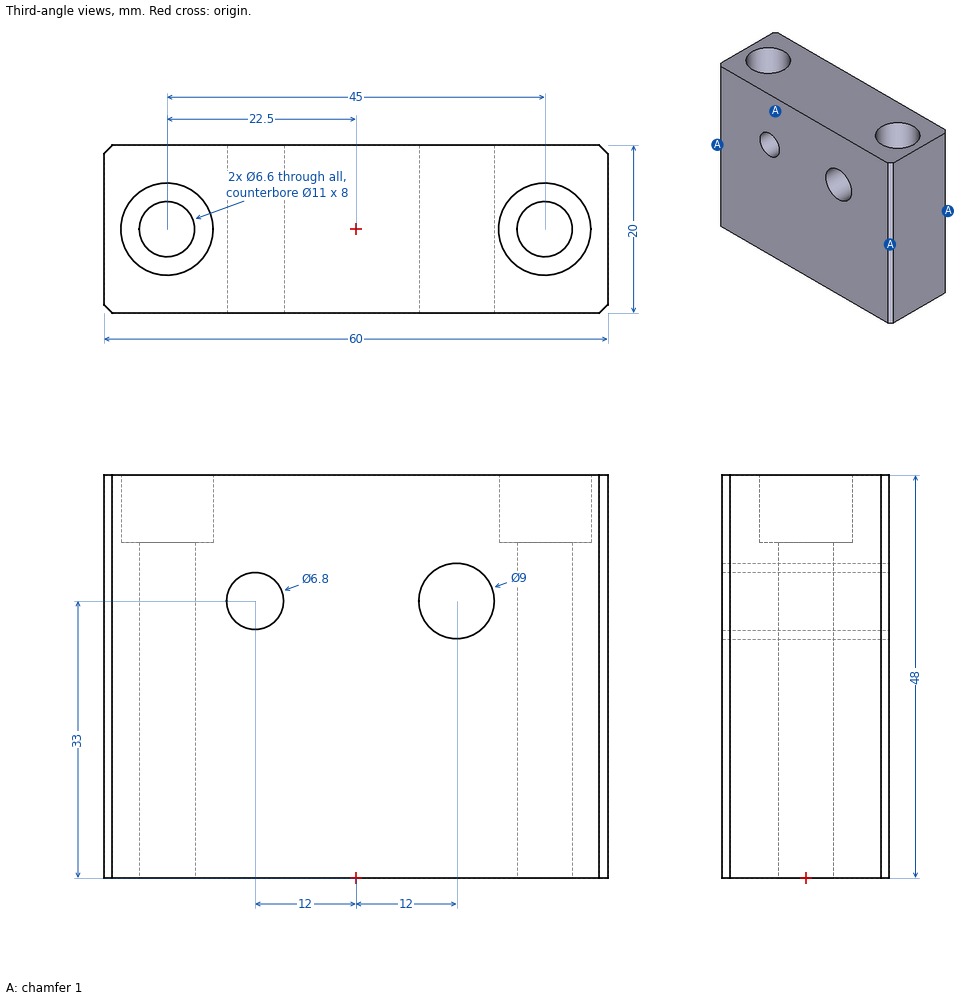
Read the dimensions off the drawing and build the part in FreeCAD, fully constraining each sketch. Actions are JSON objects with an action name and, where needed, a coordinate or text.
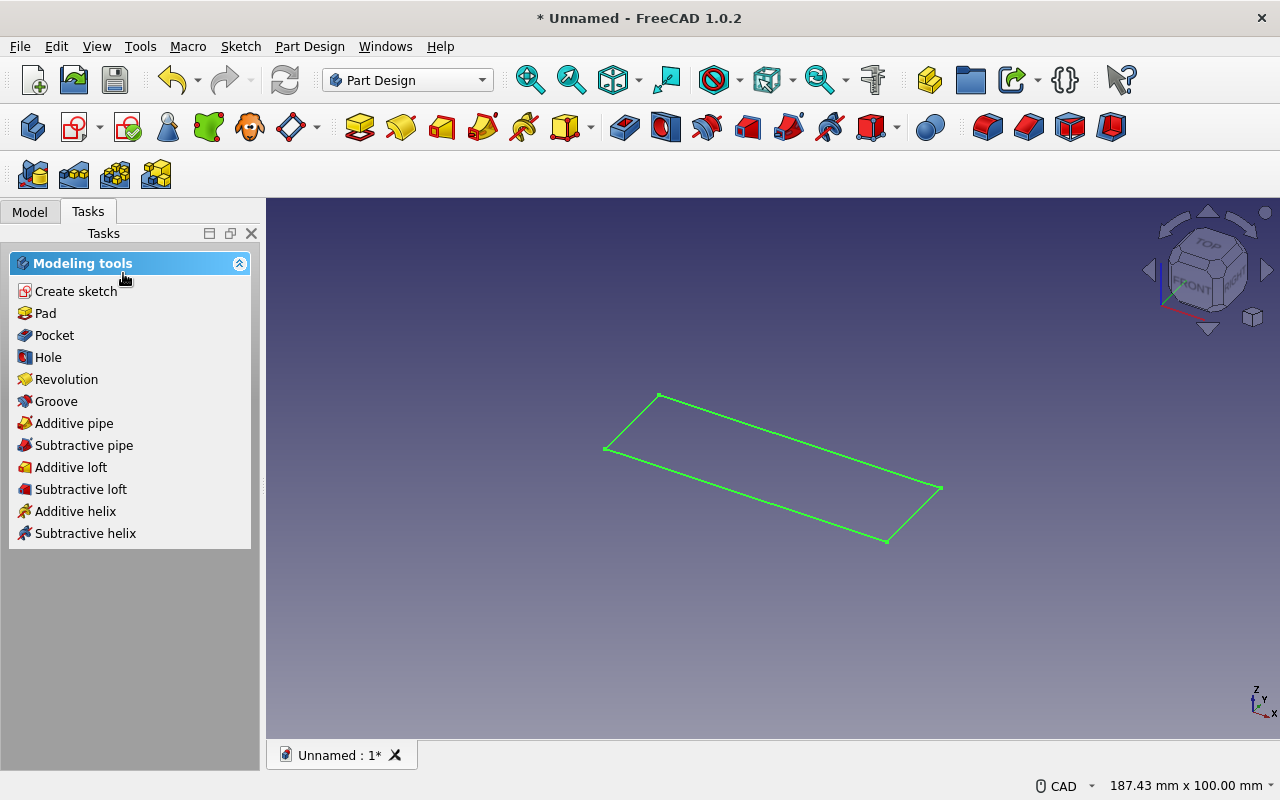
{"action": "left_click", "coordinate": [360, 128]}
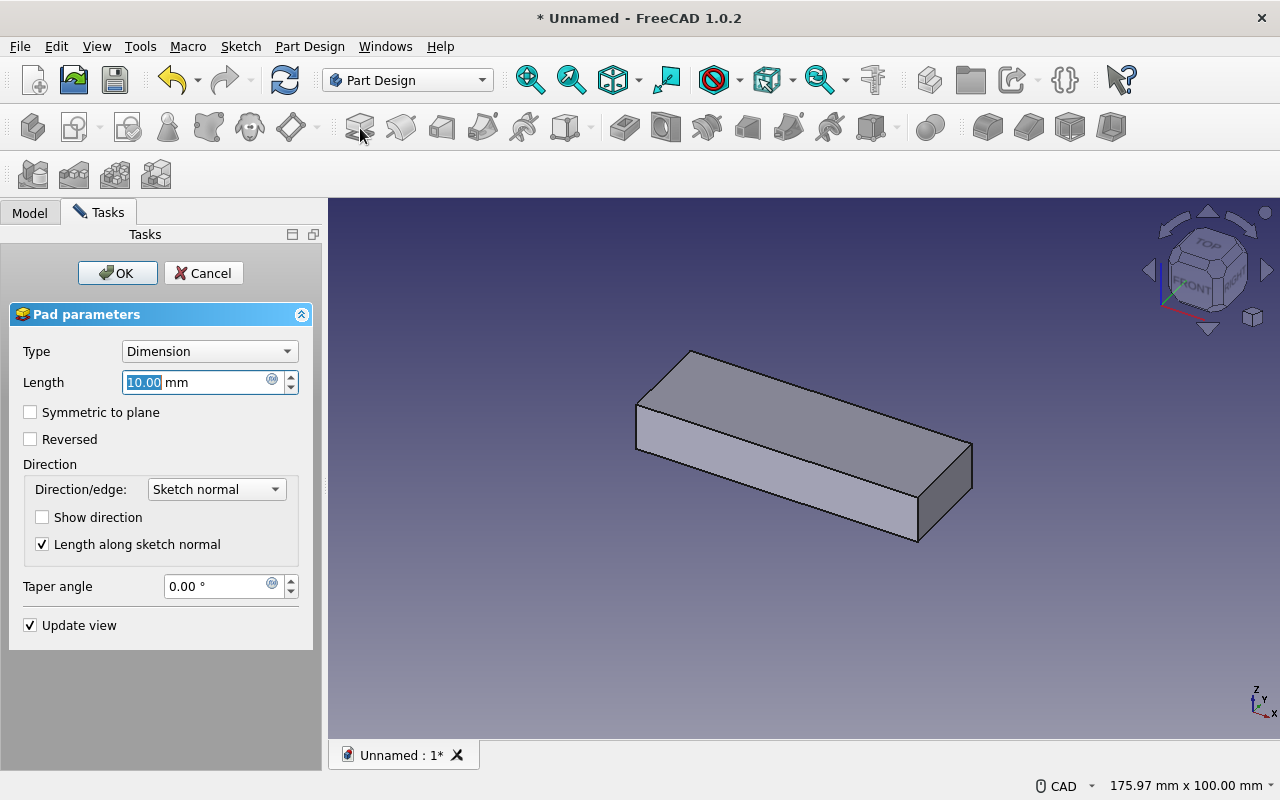
{"action": "type", "text": "48"}
{"action": "key", "text": "Tab"}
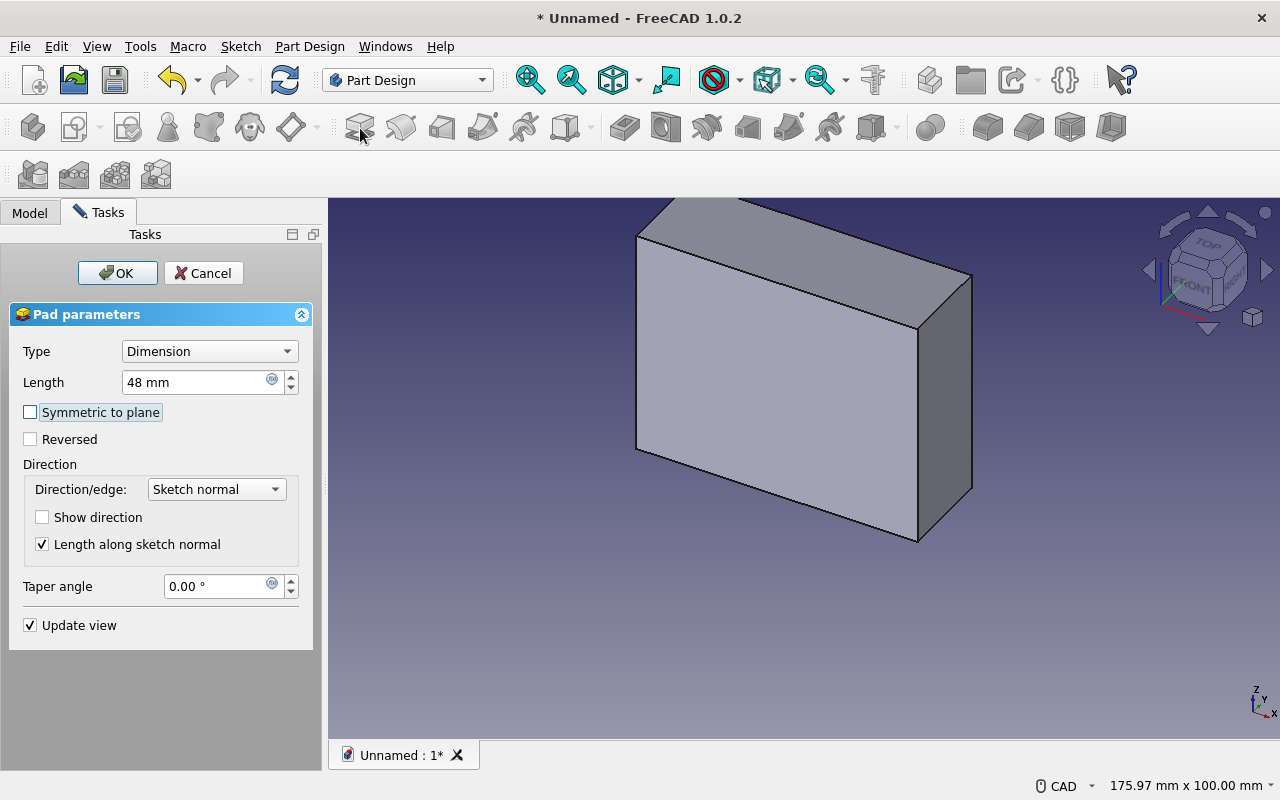
{"action": "left_click", "coordinate": [118, 273]}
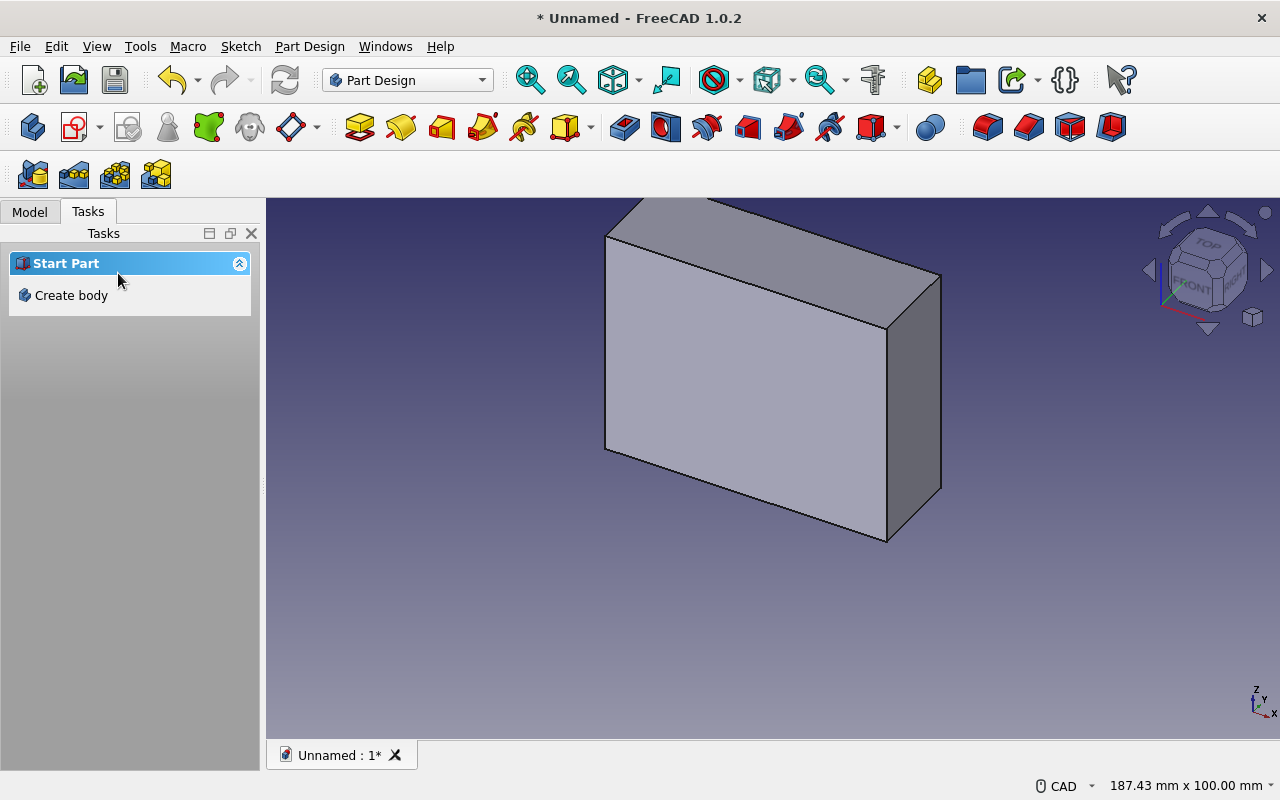
{"action": "left_click", "coordinate": [531, 80]}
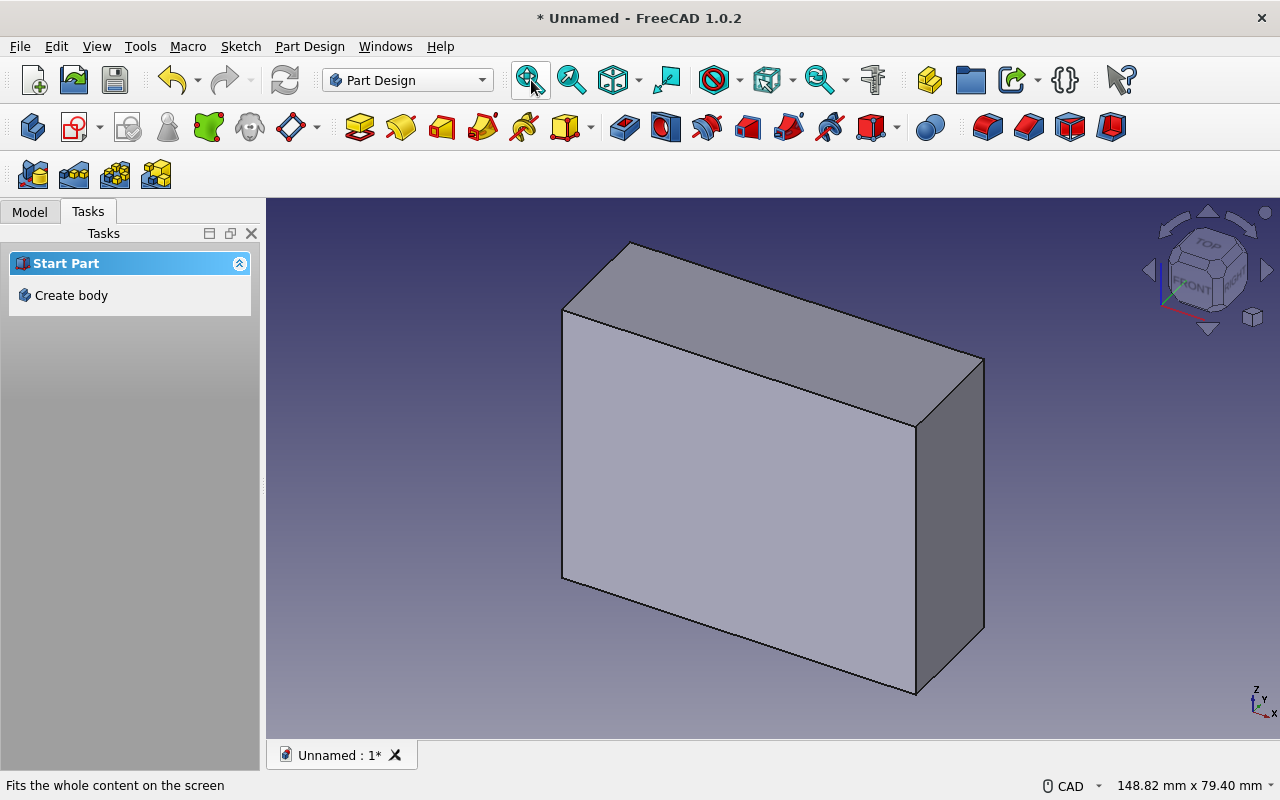
{"action": "left_click", "coordinate": [874, 367]}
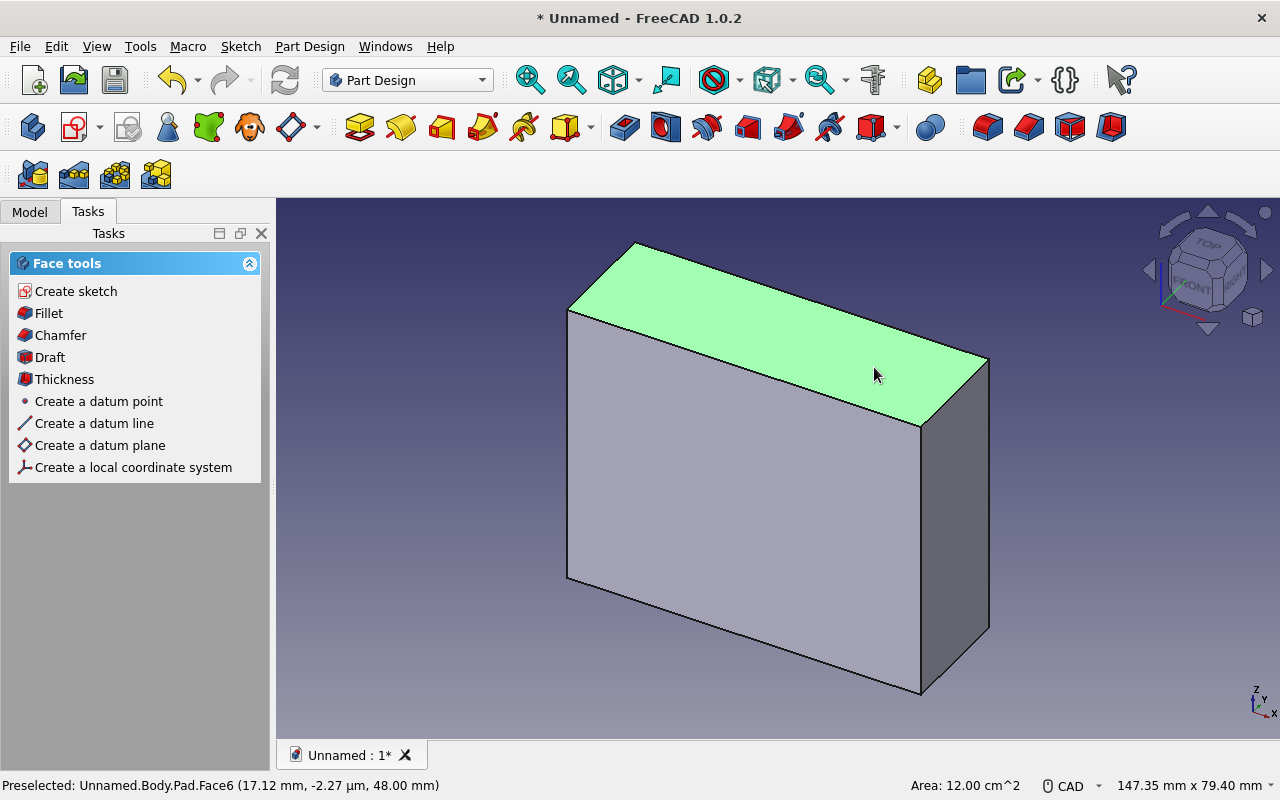
{"action": "left_click", "coordinate": [74, 128]}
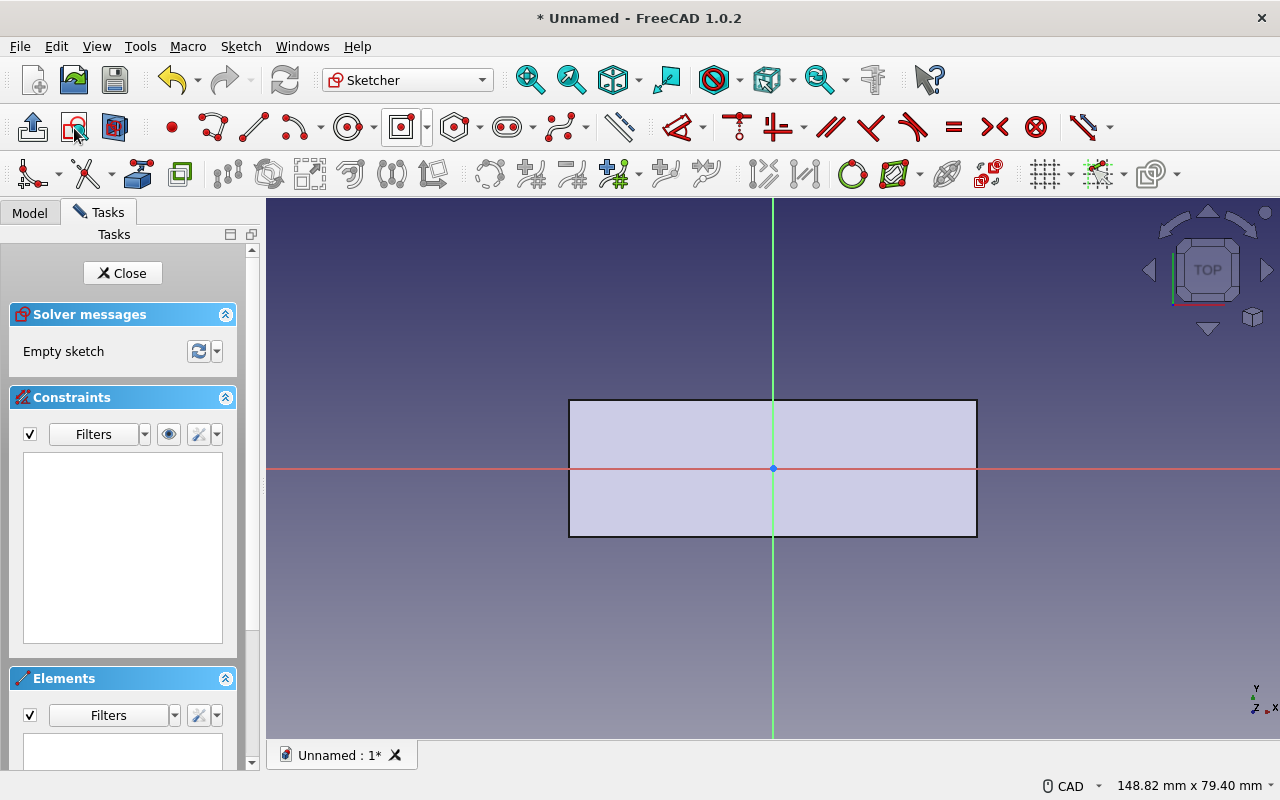
{"action": "scroll", "coordinate": [912, 469], "scroll_direction": "up", "scroll_amount": 2}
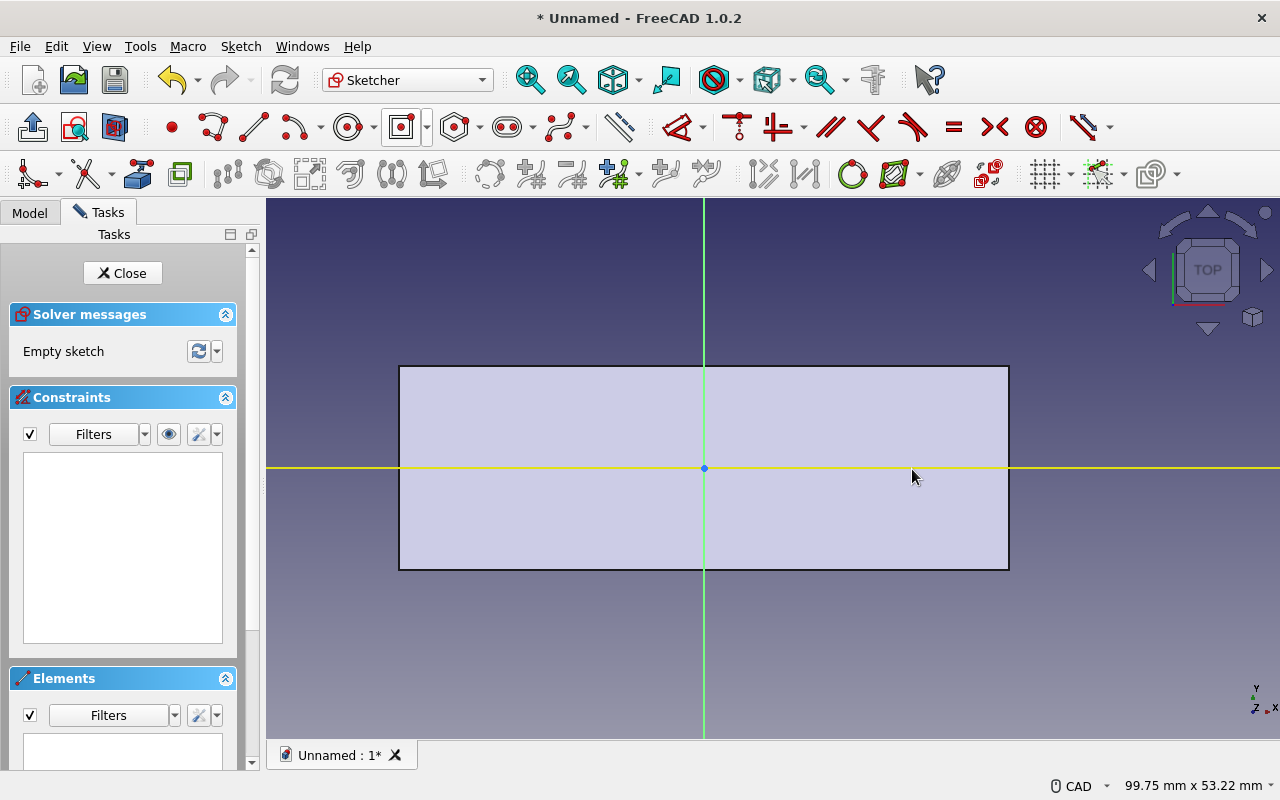
{"action": "left_click", "coordinate": [348, 128]}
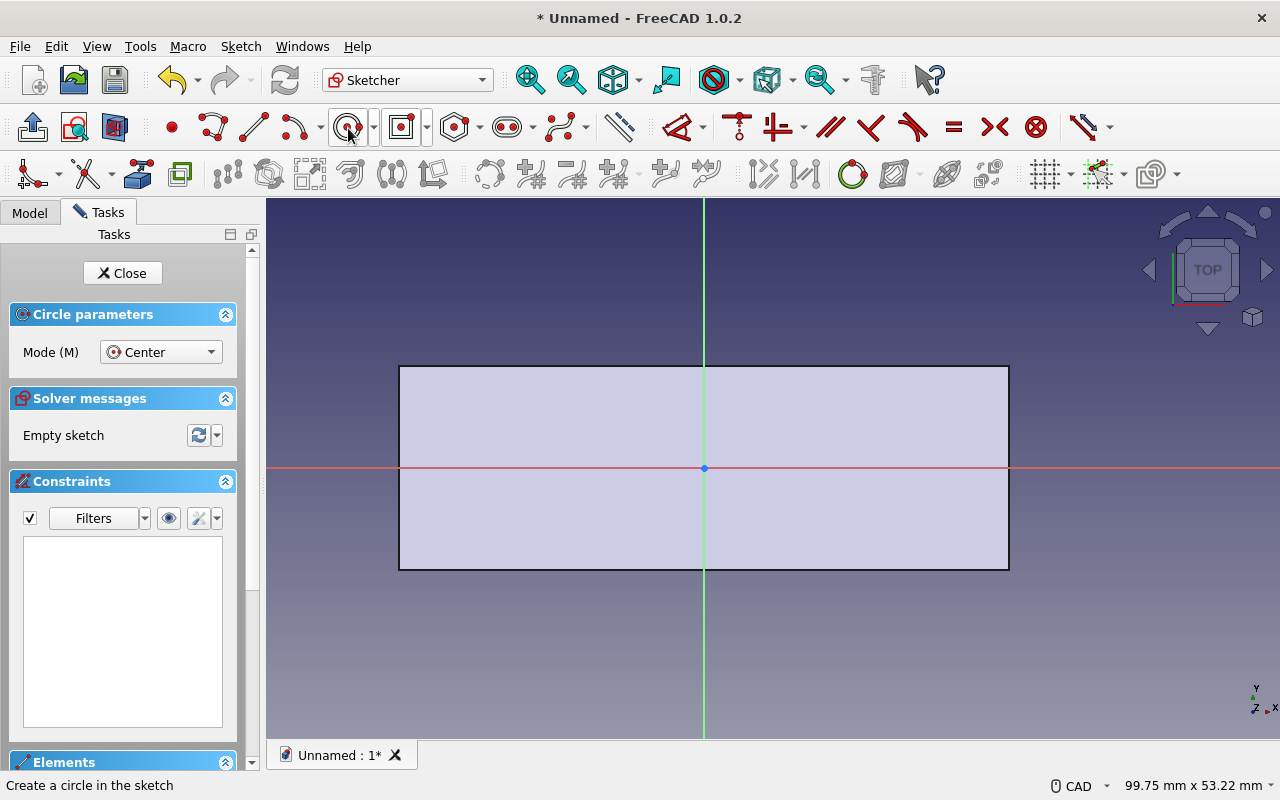
{"action": "left_click", "coordinate": [476, 468]}
{"action": "mouse_move", "coordinate": [499, 444]}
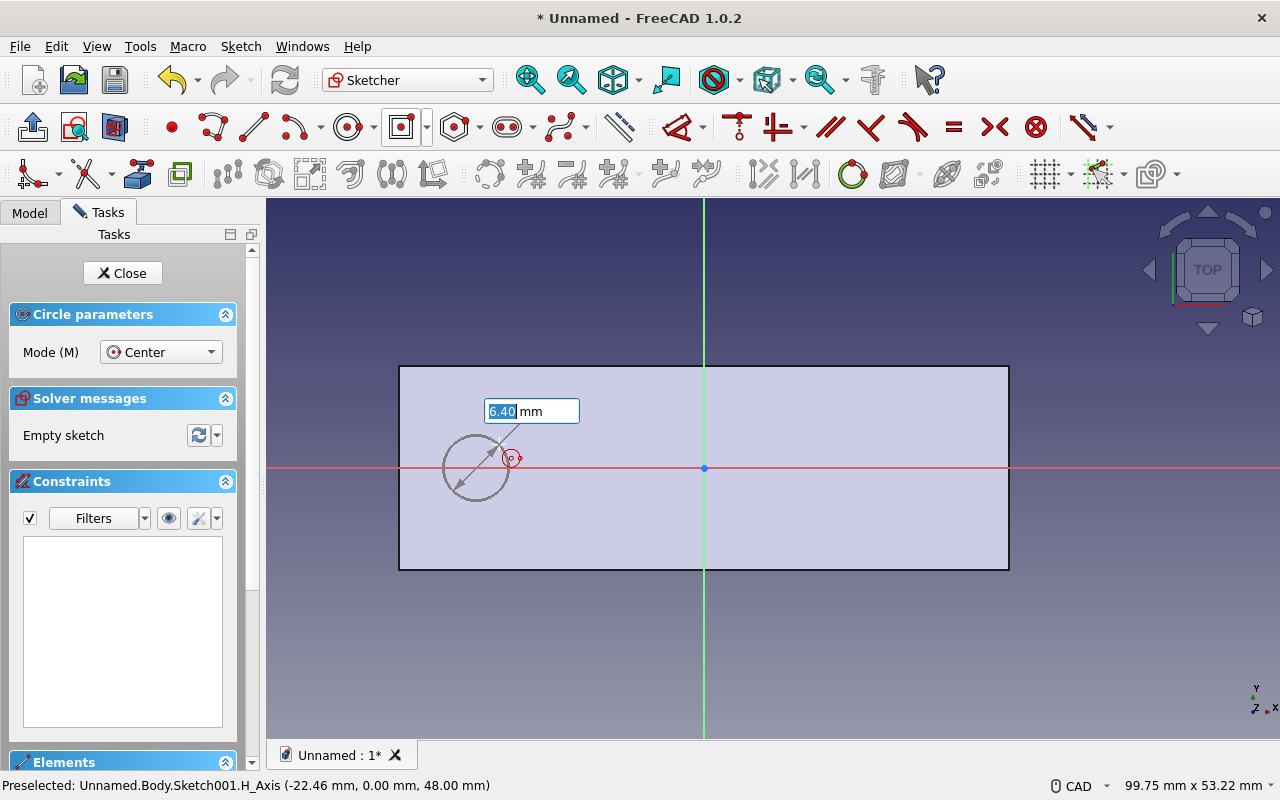
{"action": "type", "text": "6.6"}
{"action": "key", "text": "Return"}